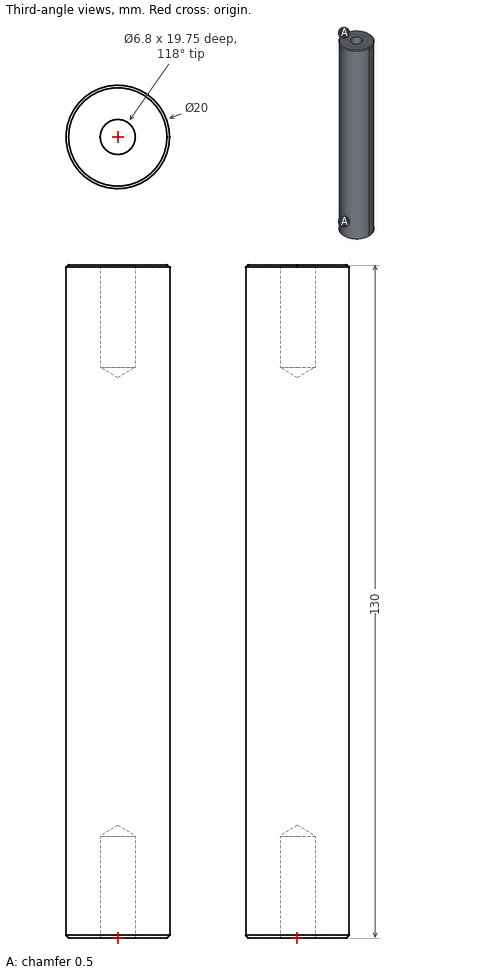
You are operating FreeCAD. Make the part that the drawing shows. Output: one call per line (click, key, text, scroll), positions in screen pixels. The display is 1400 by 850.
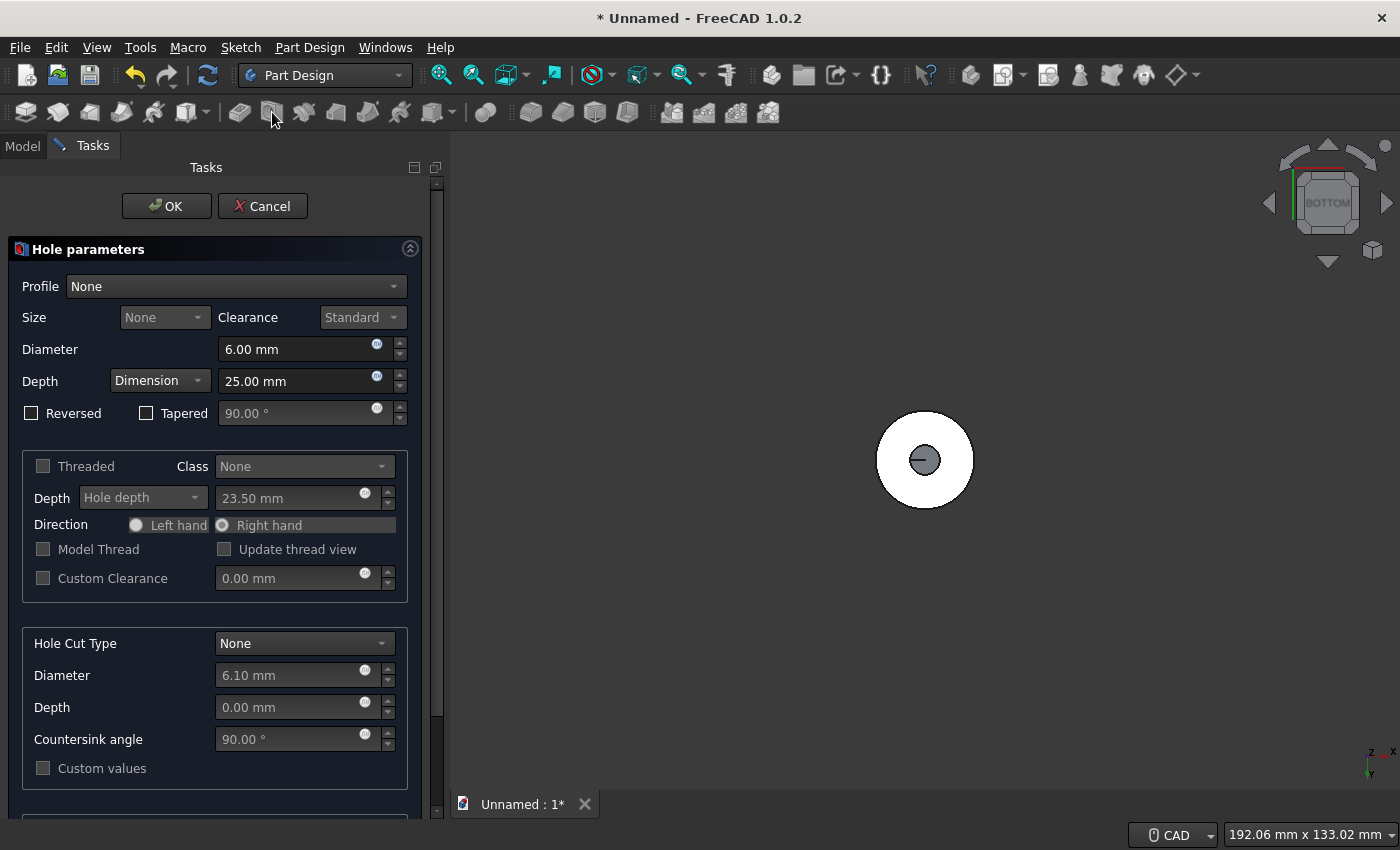
triple_click(305, 349)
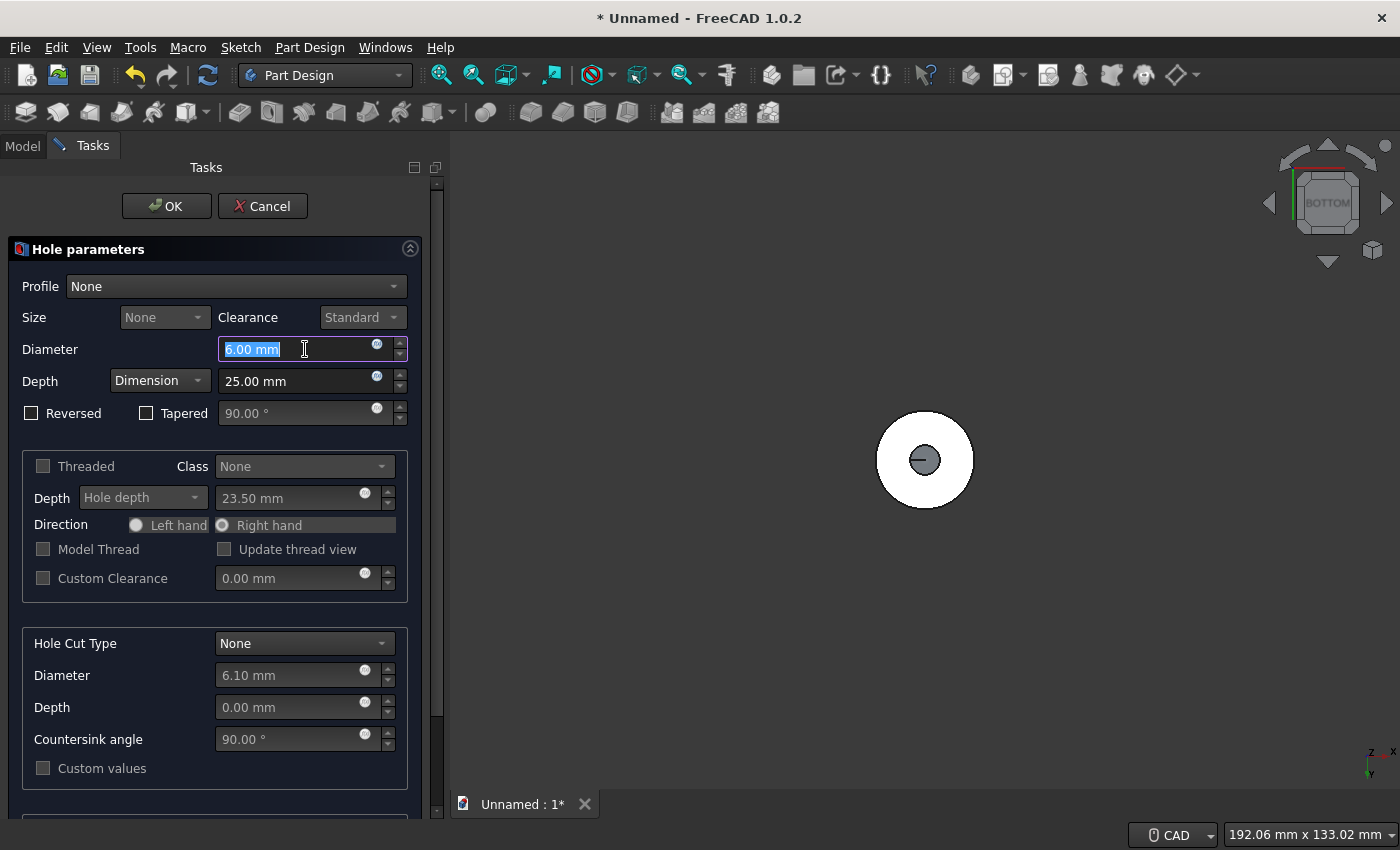
text(6.8)
key(Tab)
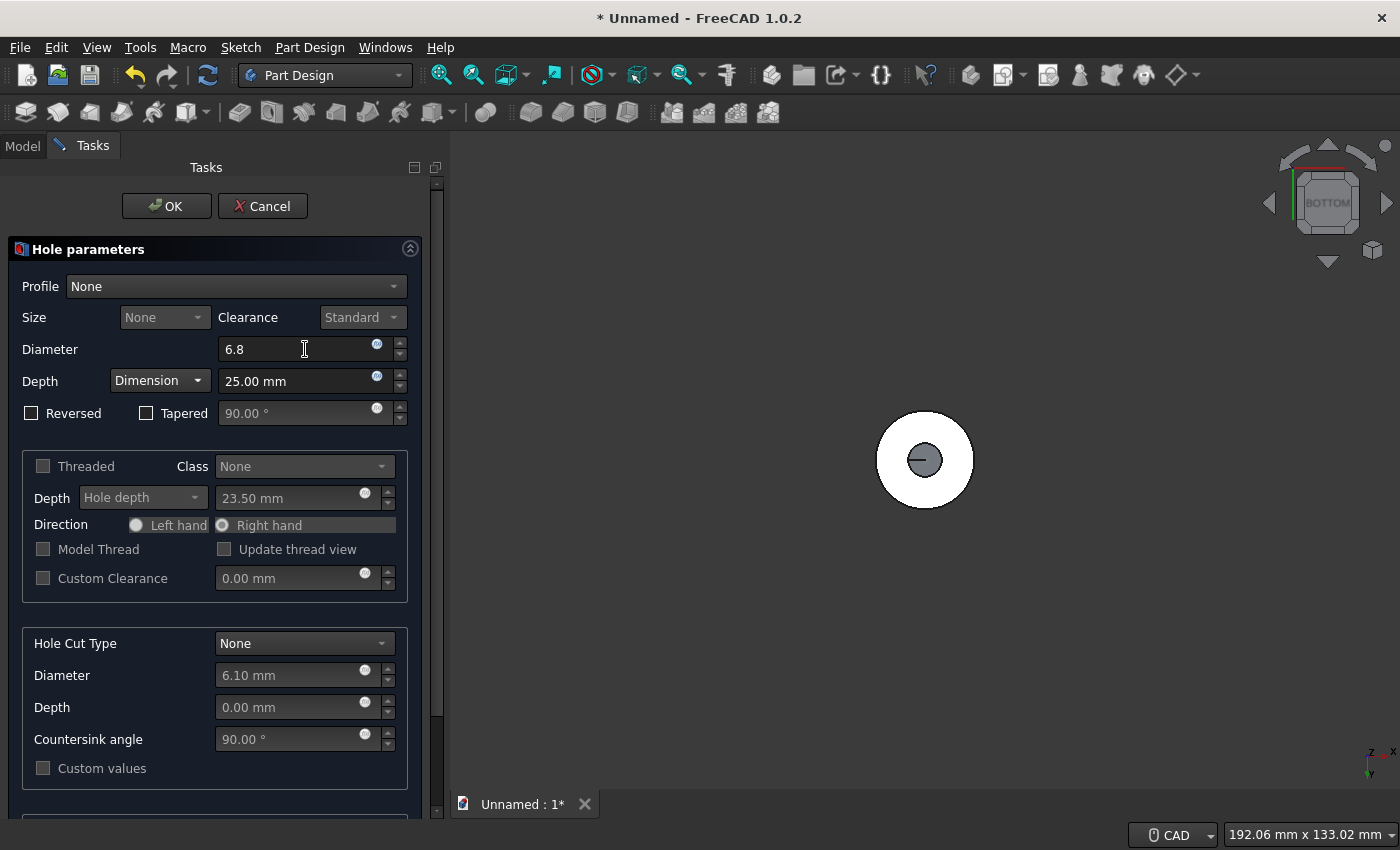
triple_click(305, 381)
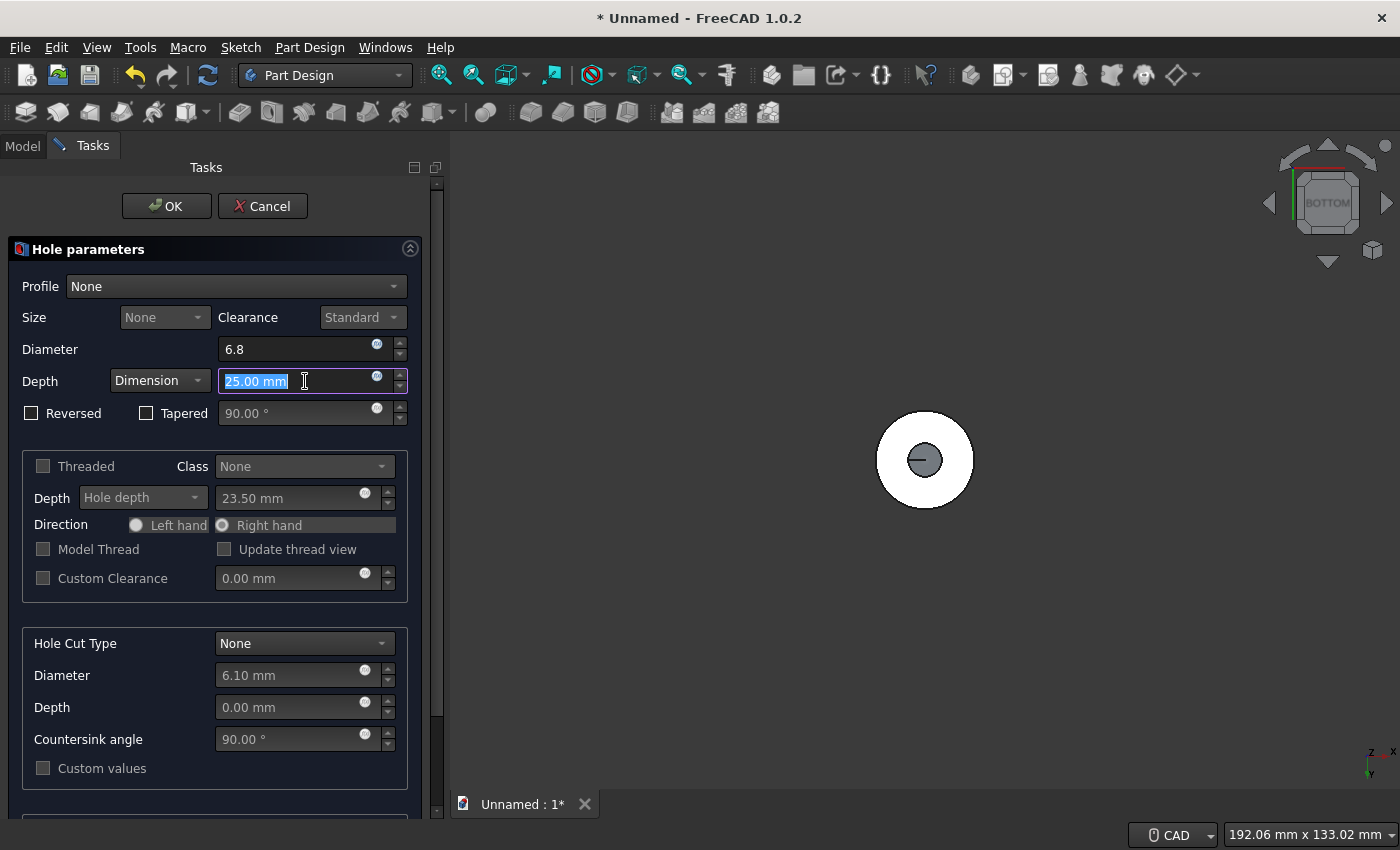
text(19.75)
key(Tab)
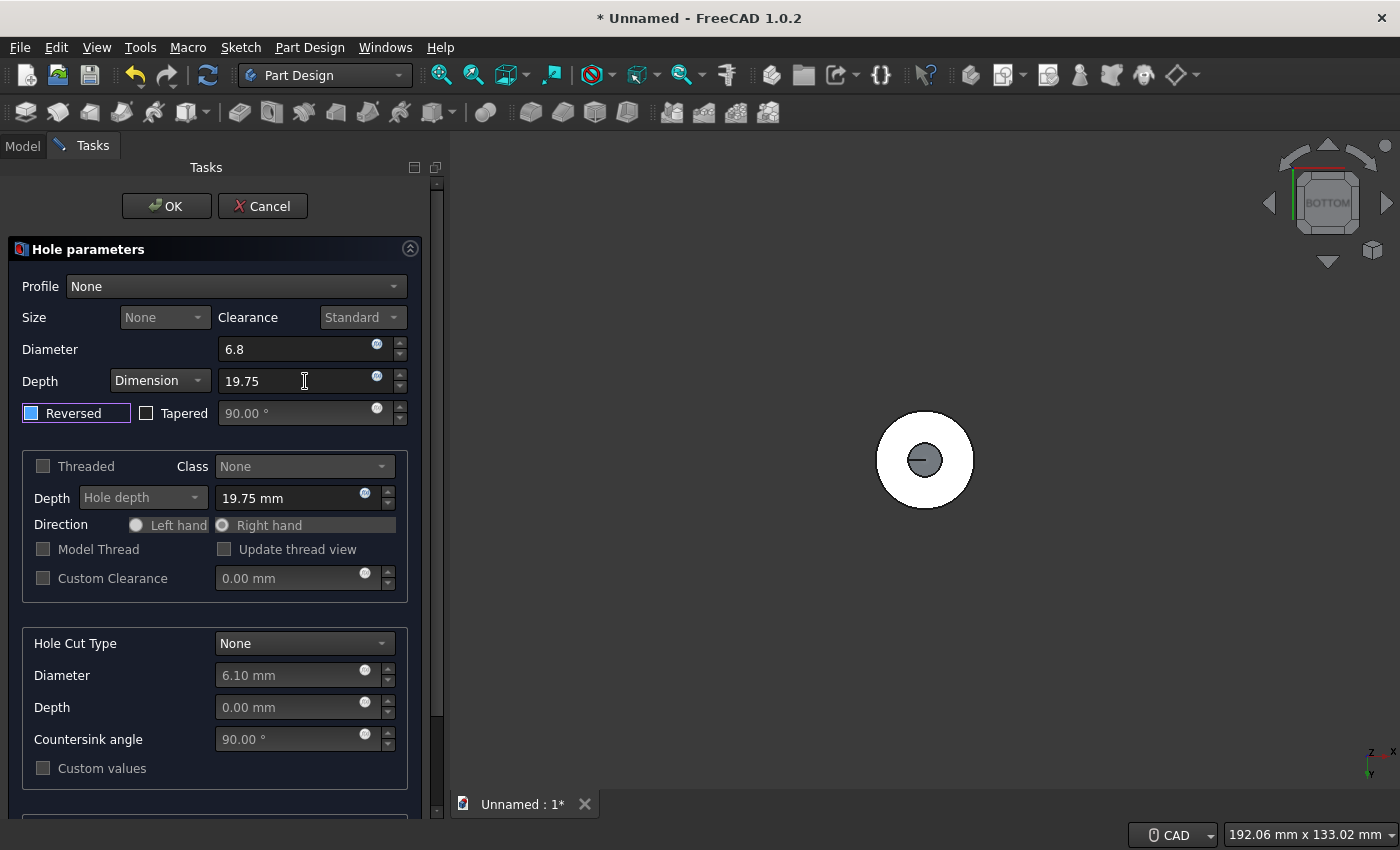
click(167, 206)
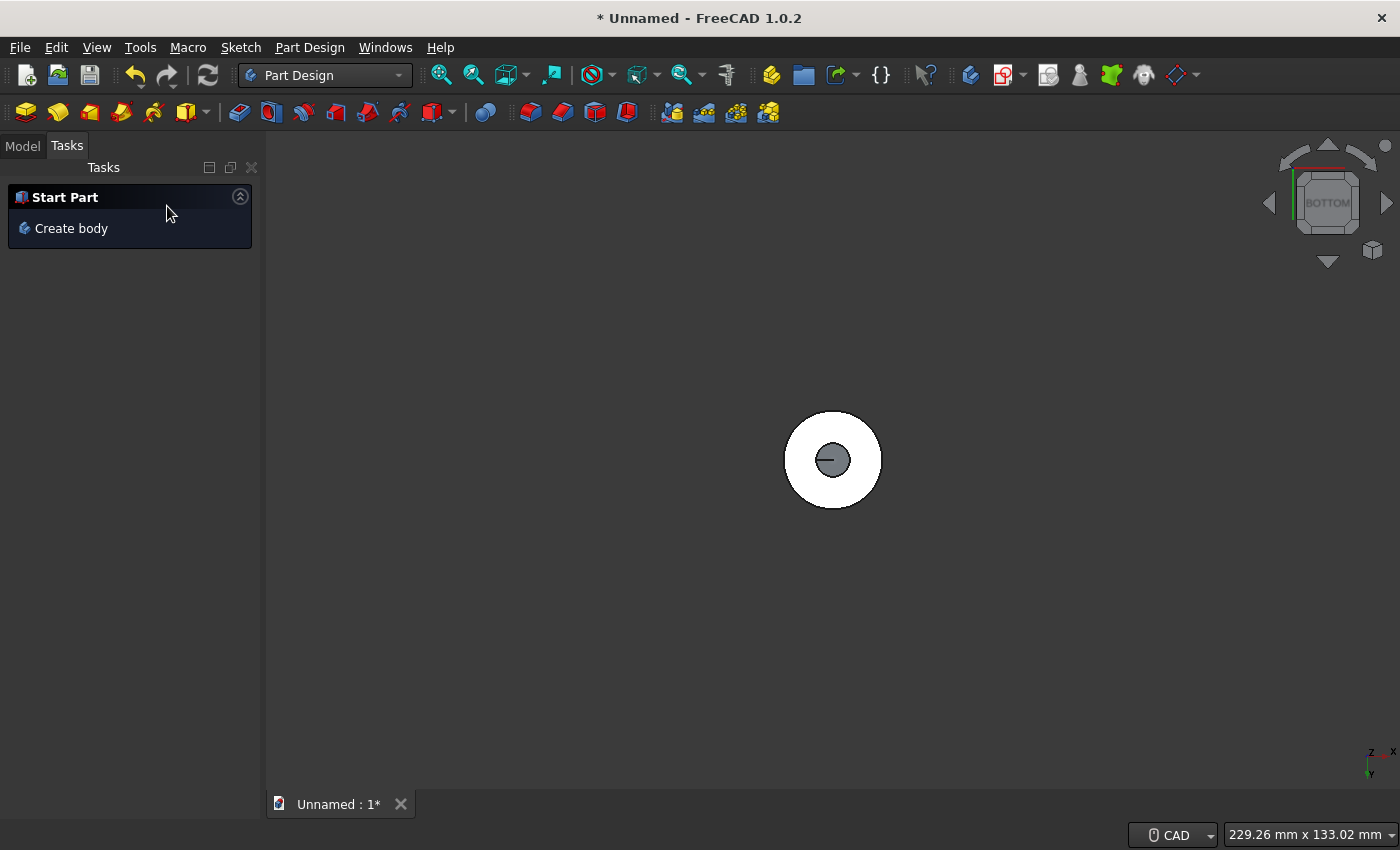
key(v)
key(f)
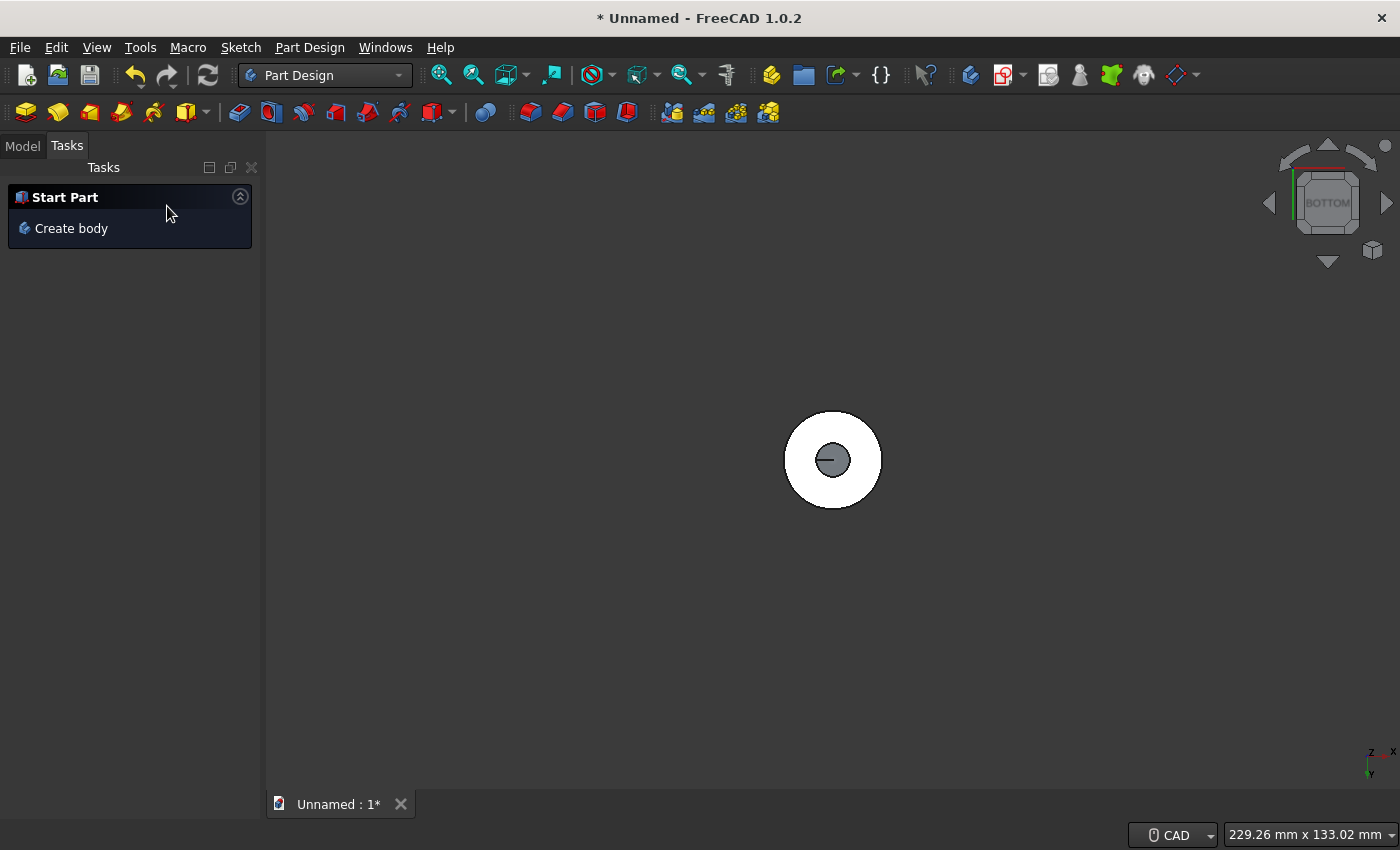
key(0)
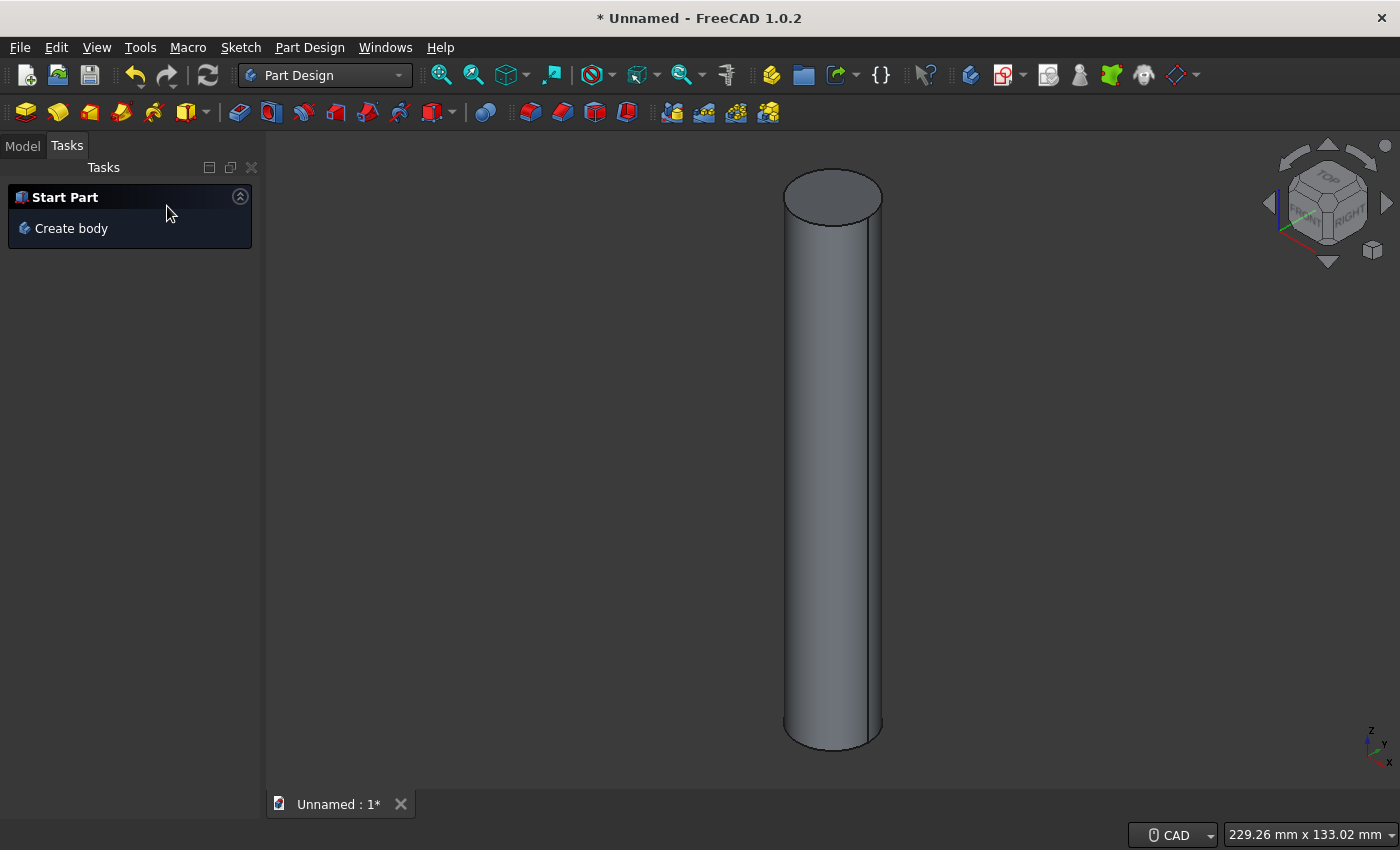
click(833, 196)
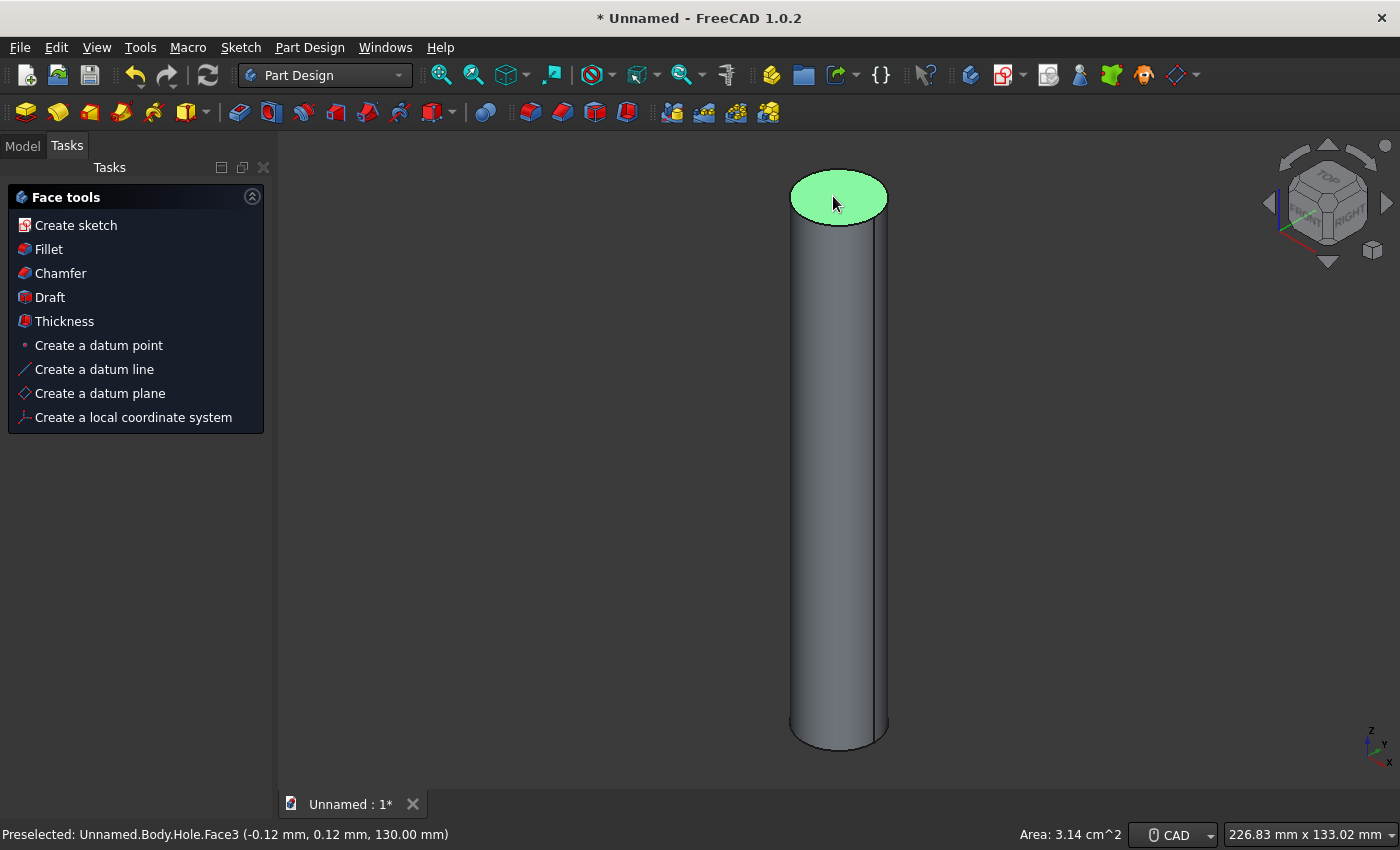
click(1004, 76)